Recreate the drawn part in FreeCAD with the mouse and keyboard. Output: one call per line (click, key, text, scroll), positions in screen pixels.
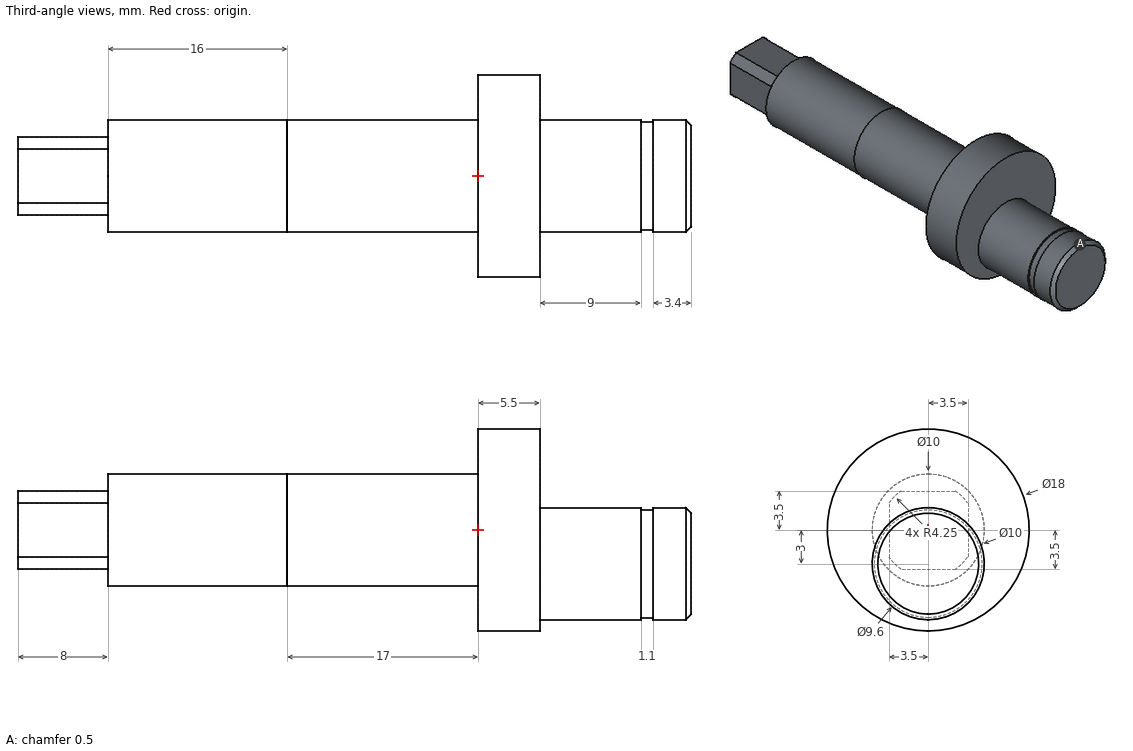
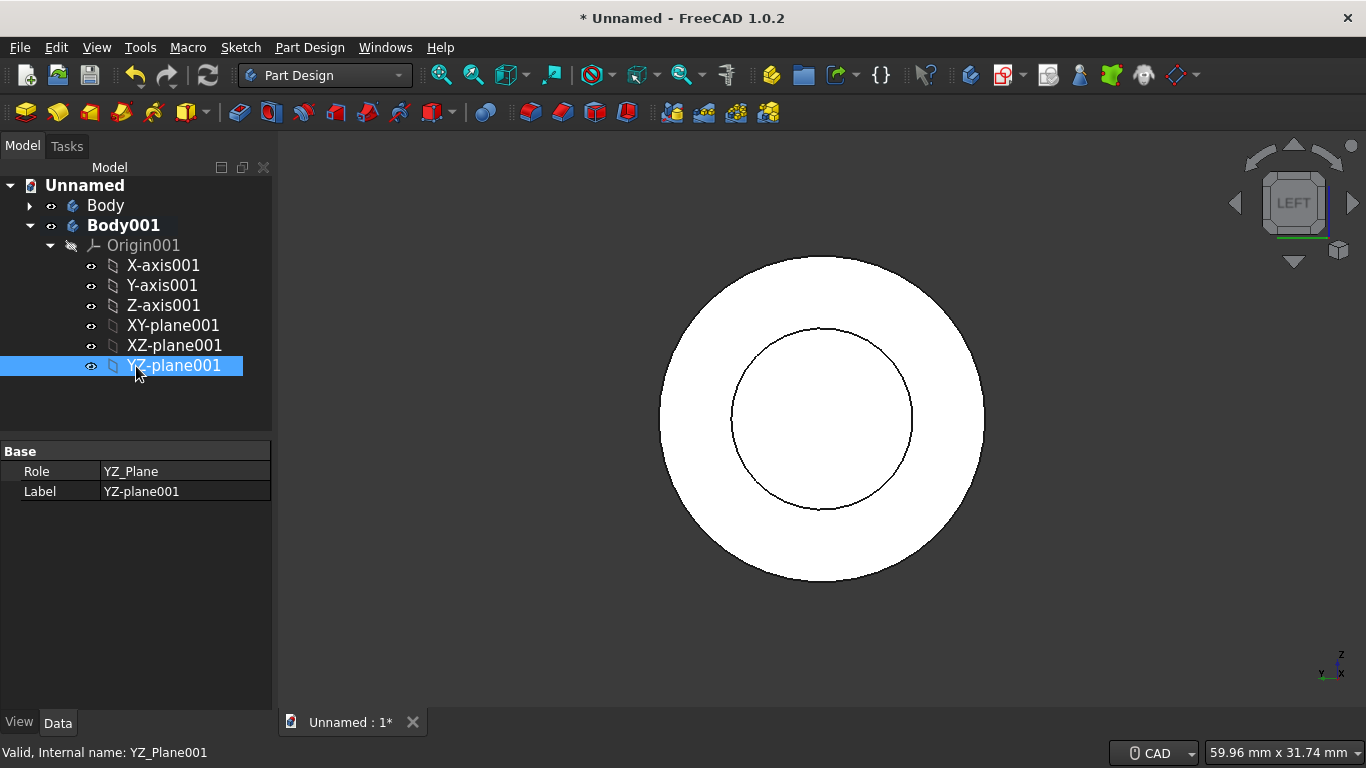
click(1176, 76)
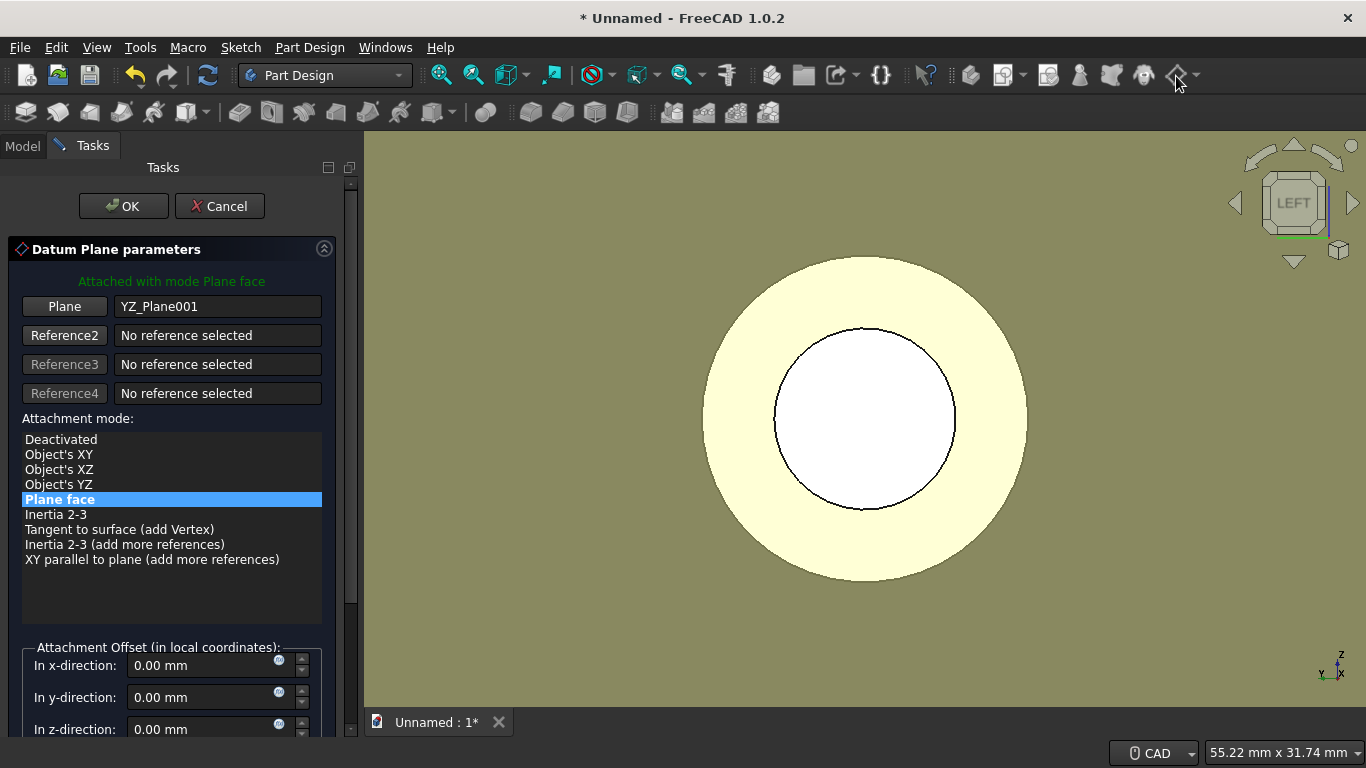
scroll(351, 456, down, 2)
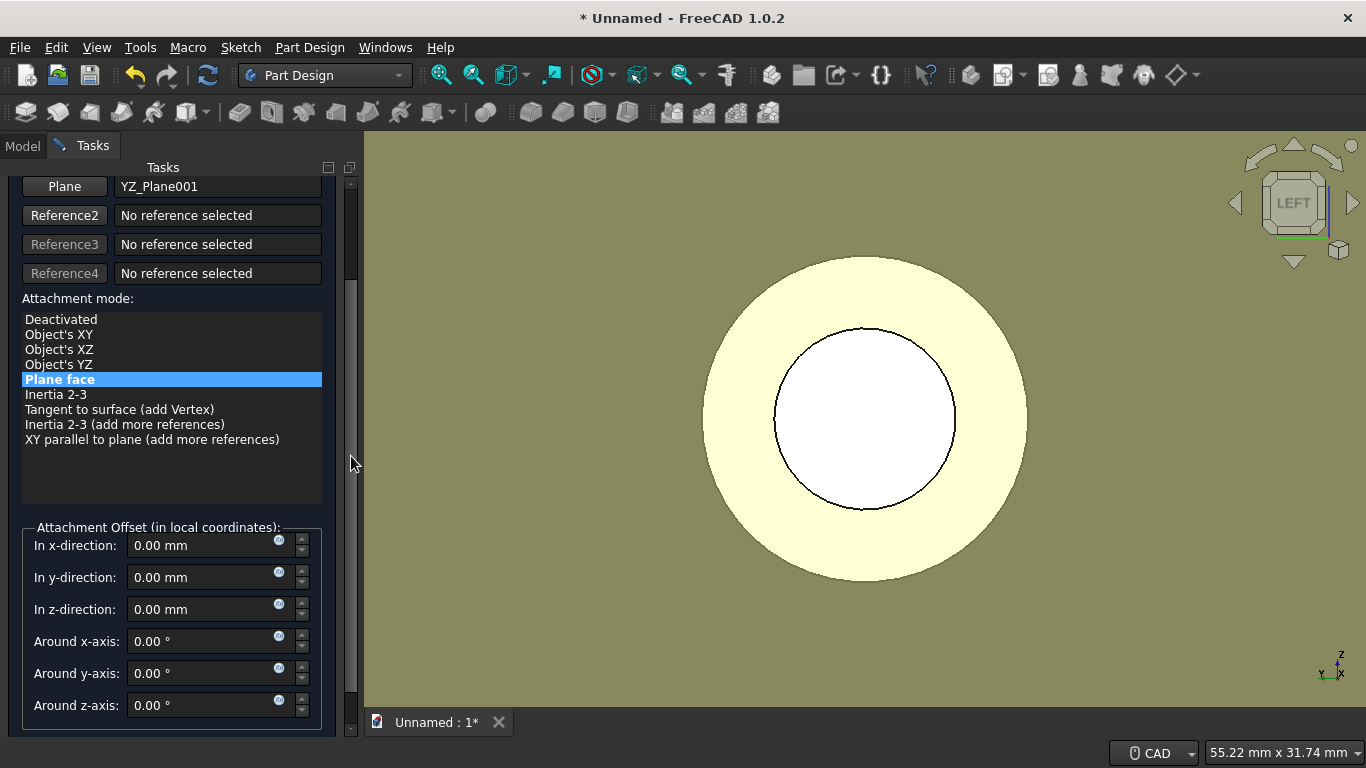
triple_click(210, 609)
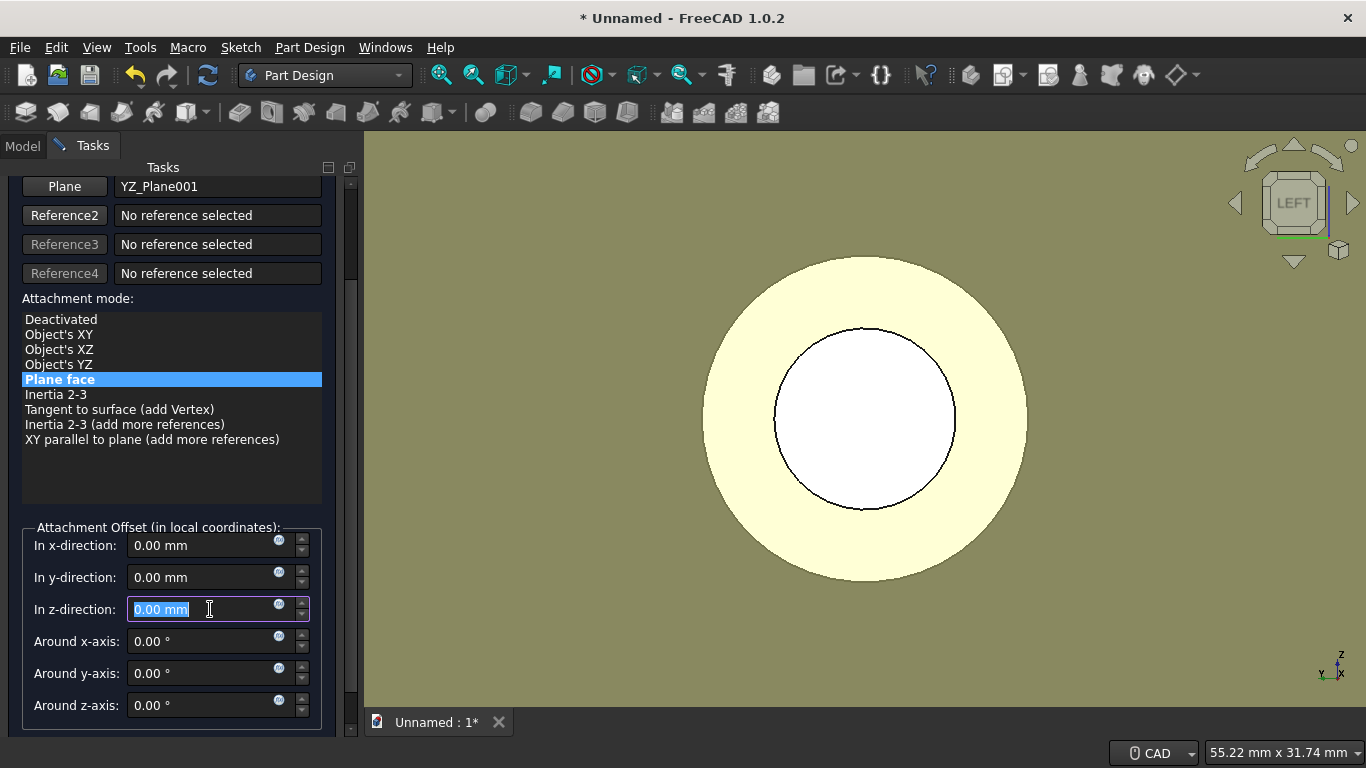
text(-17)
key(Tab)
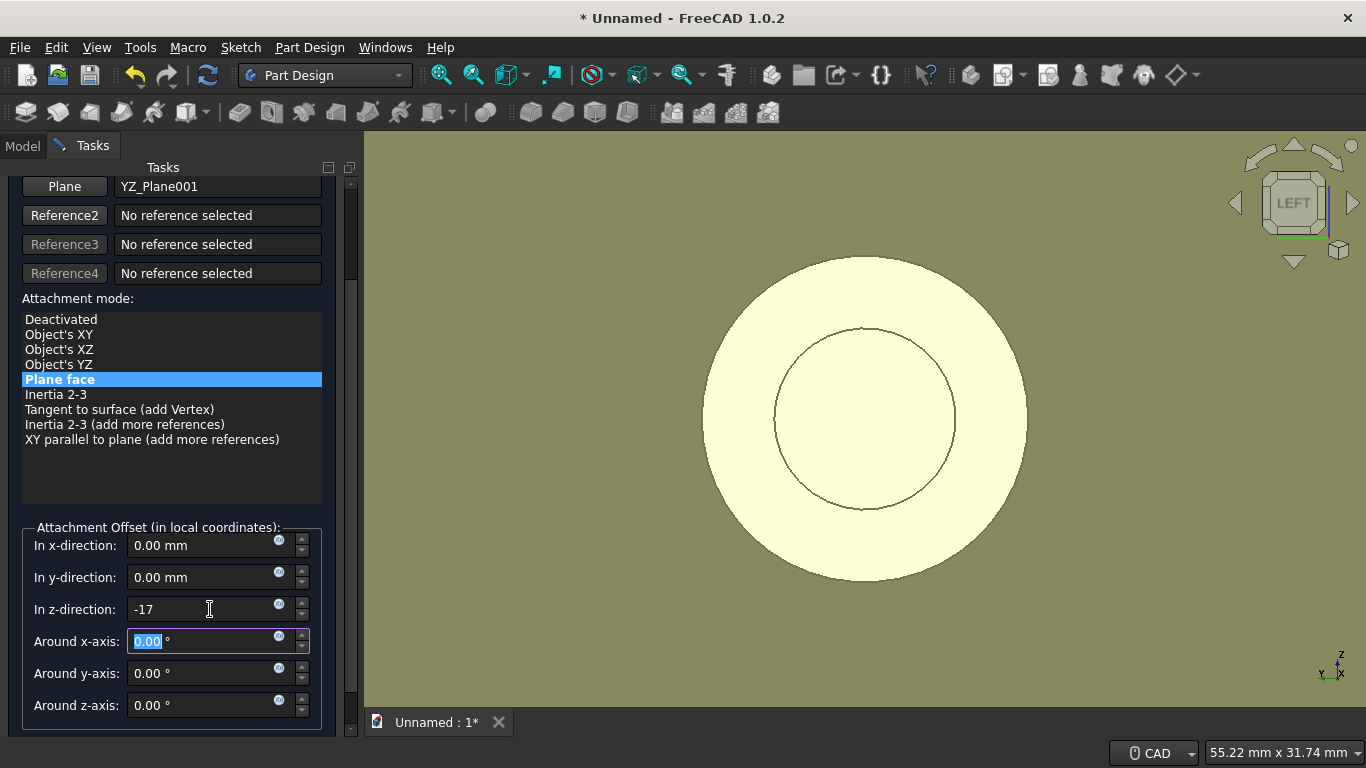
scroll(351, 456, up, 3)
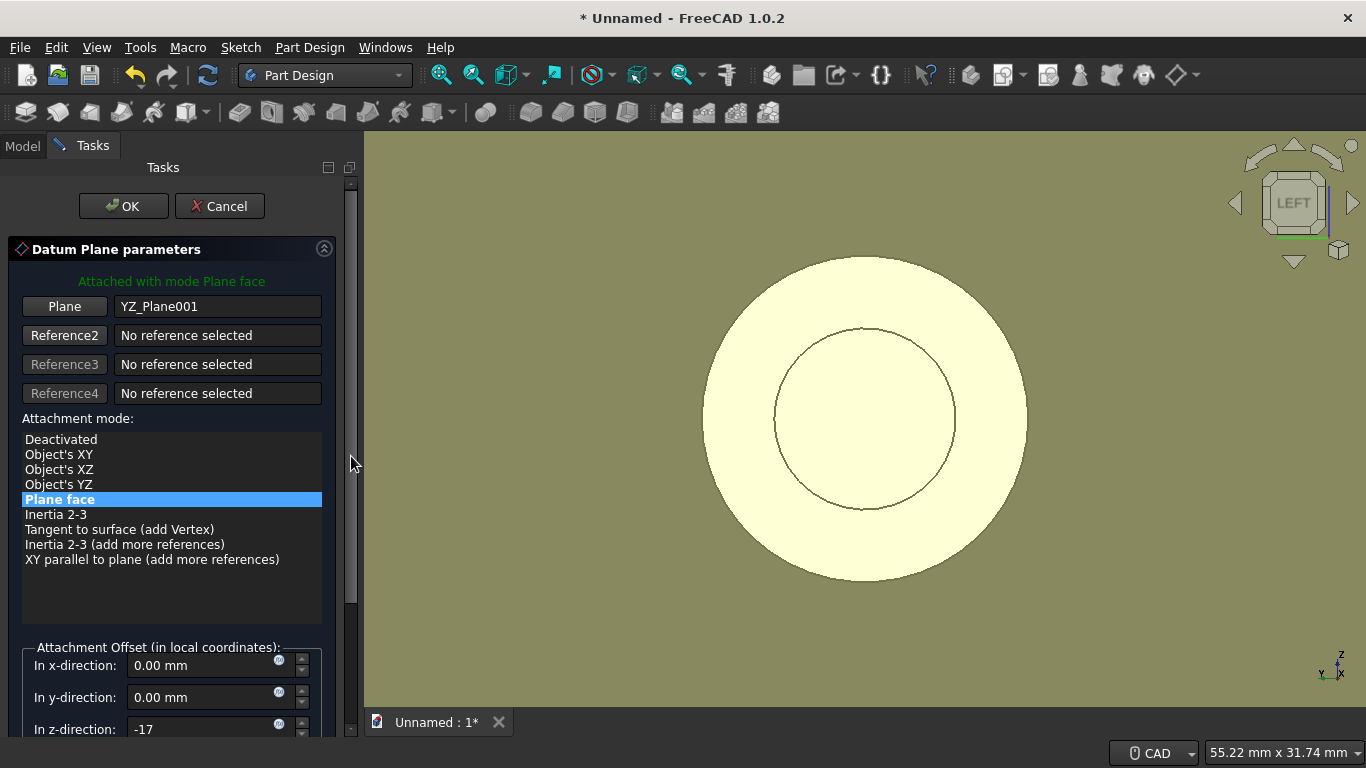
click(124, 206)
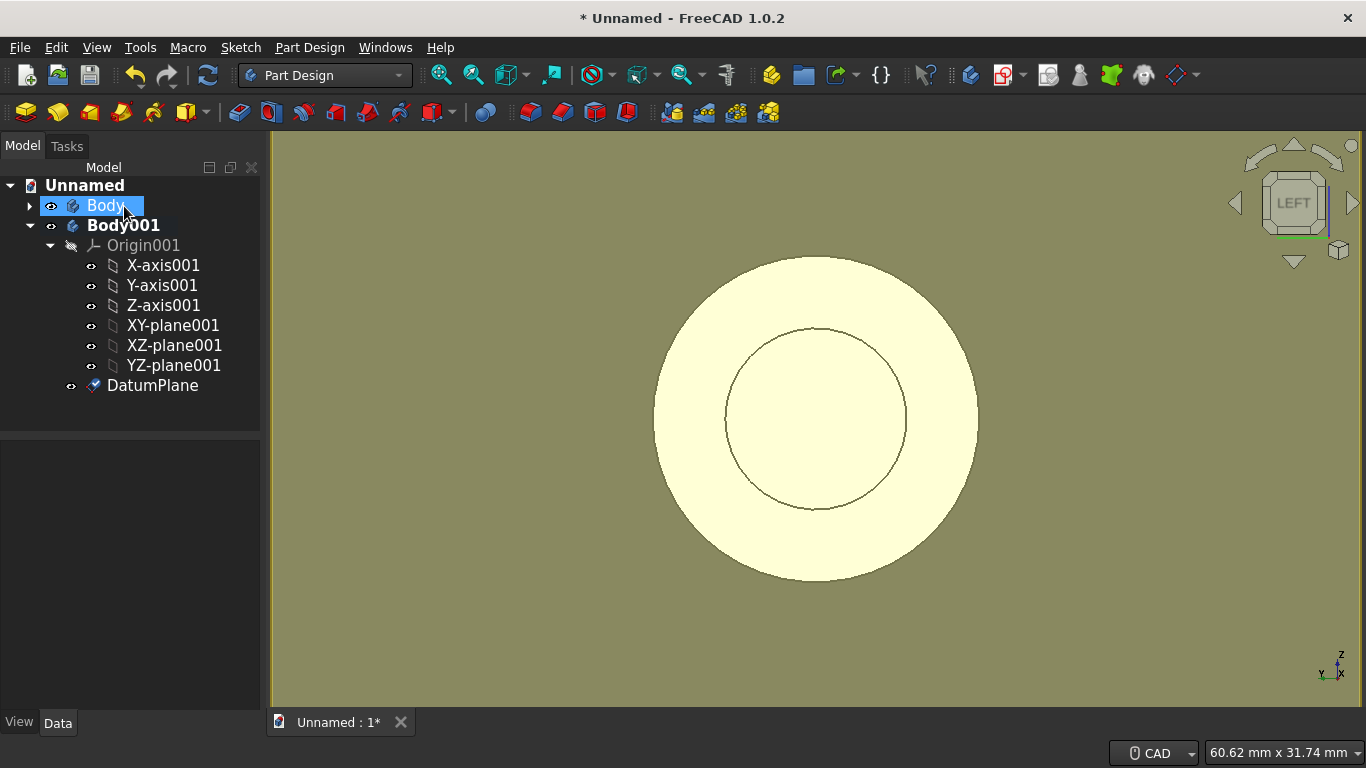
click(116, 386)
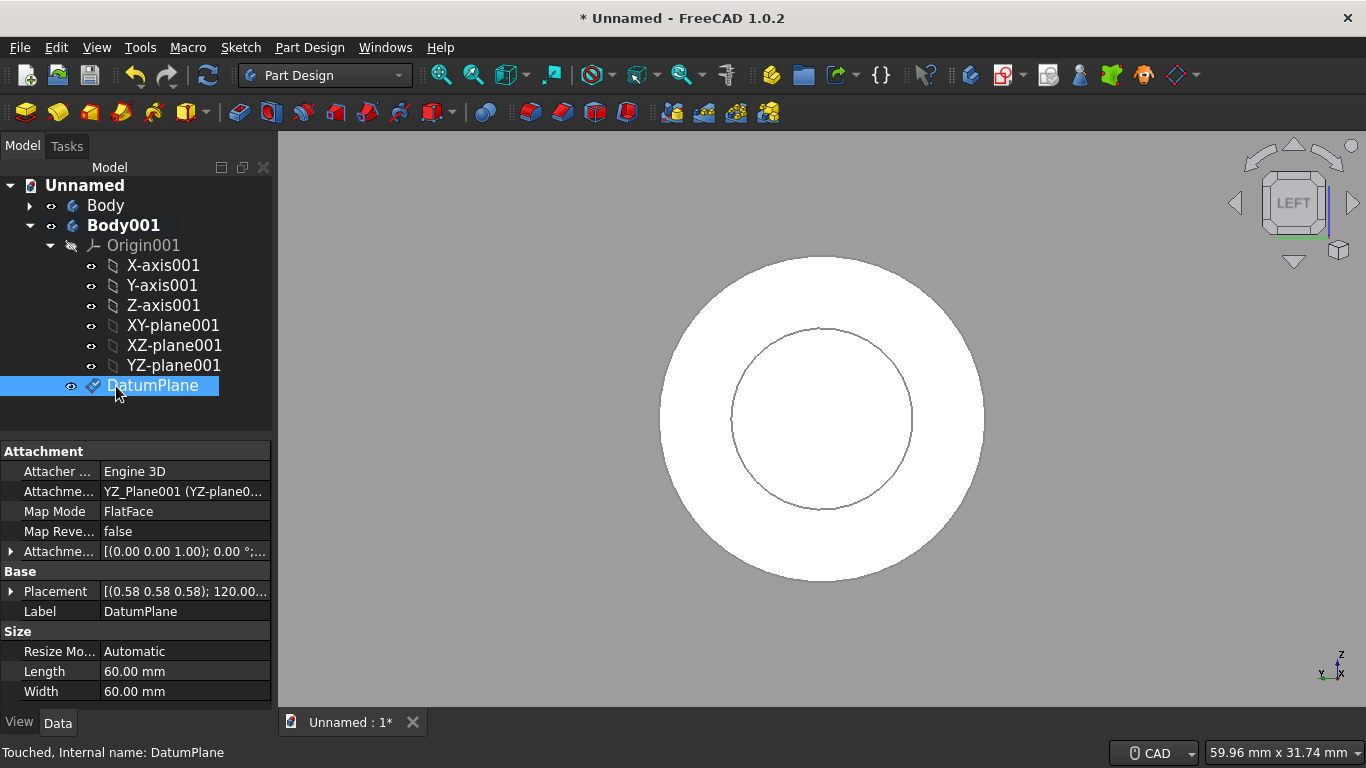
click(1004, 76)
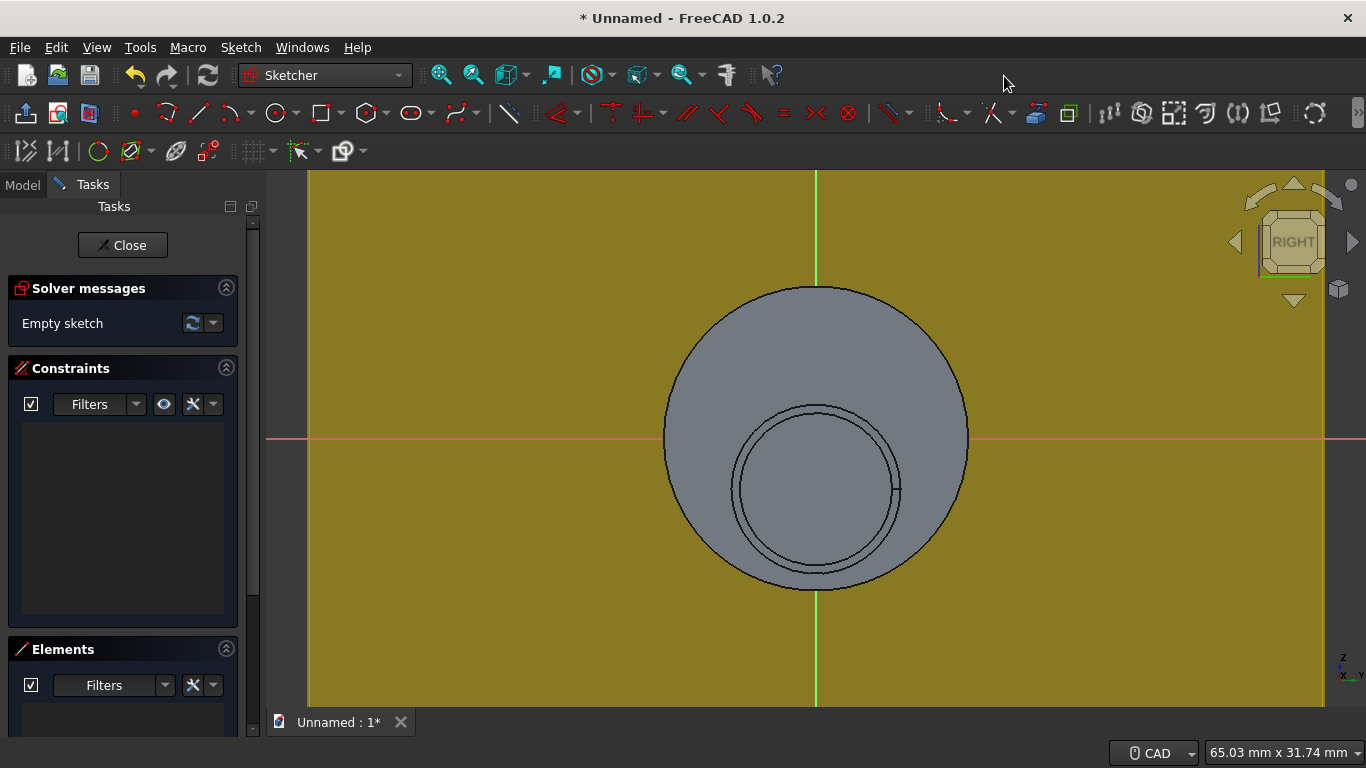
scroll(899, 439, up, 3)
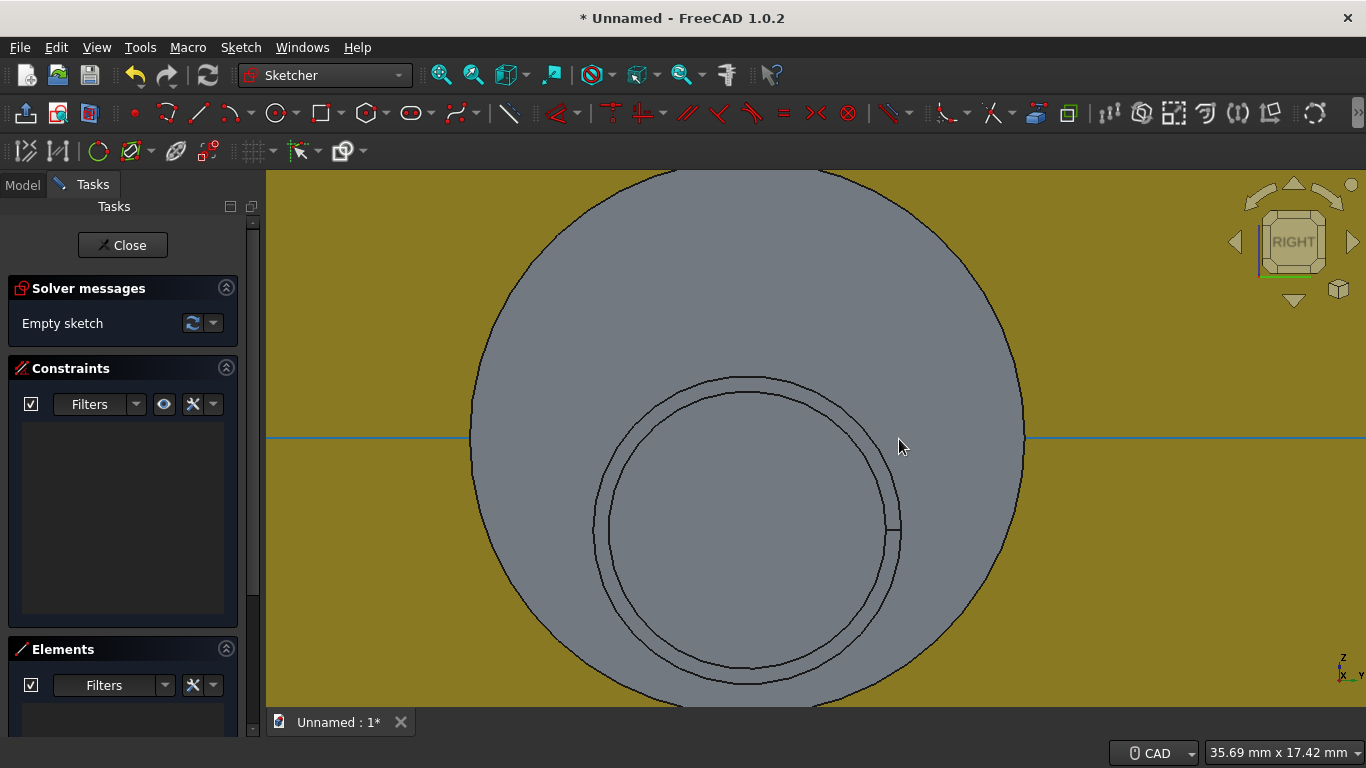
click(276, 114)